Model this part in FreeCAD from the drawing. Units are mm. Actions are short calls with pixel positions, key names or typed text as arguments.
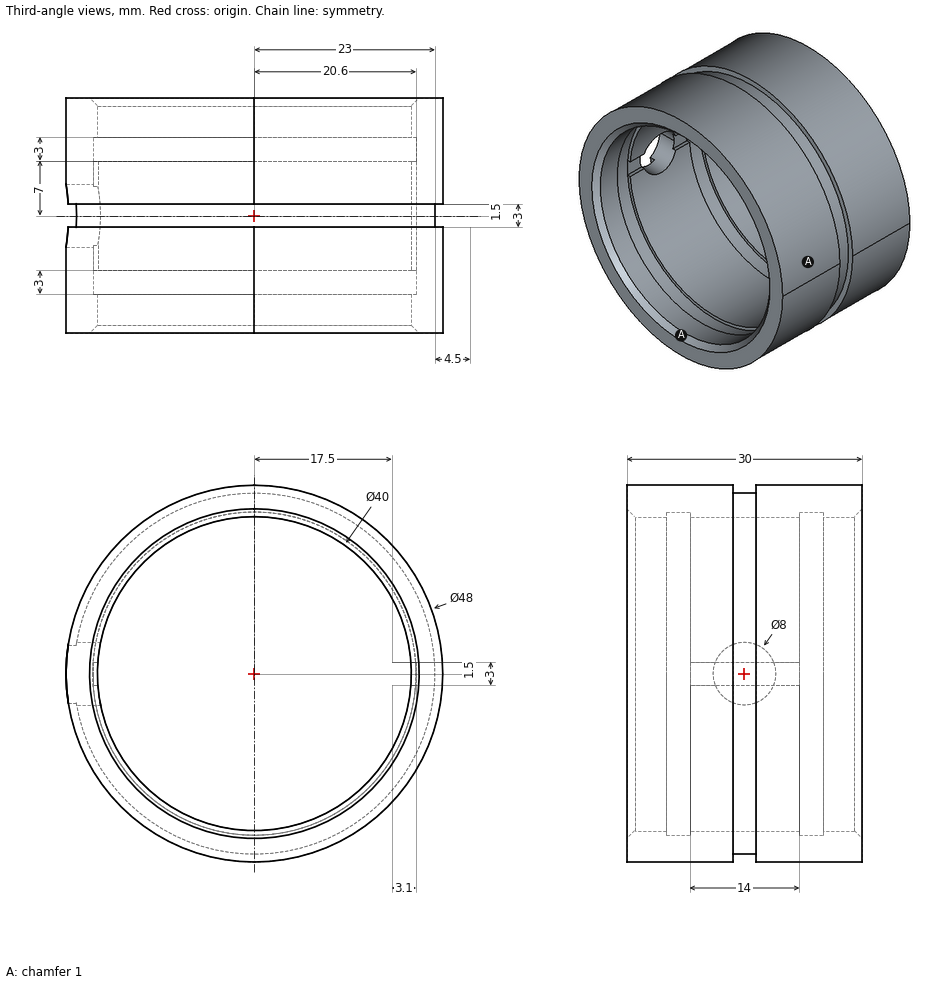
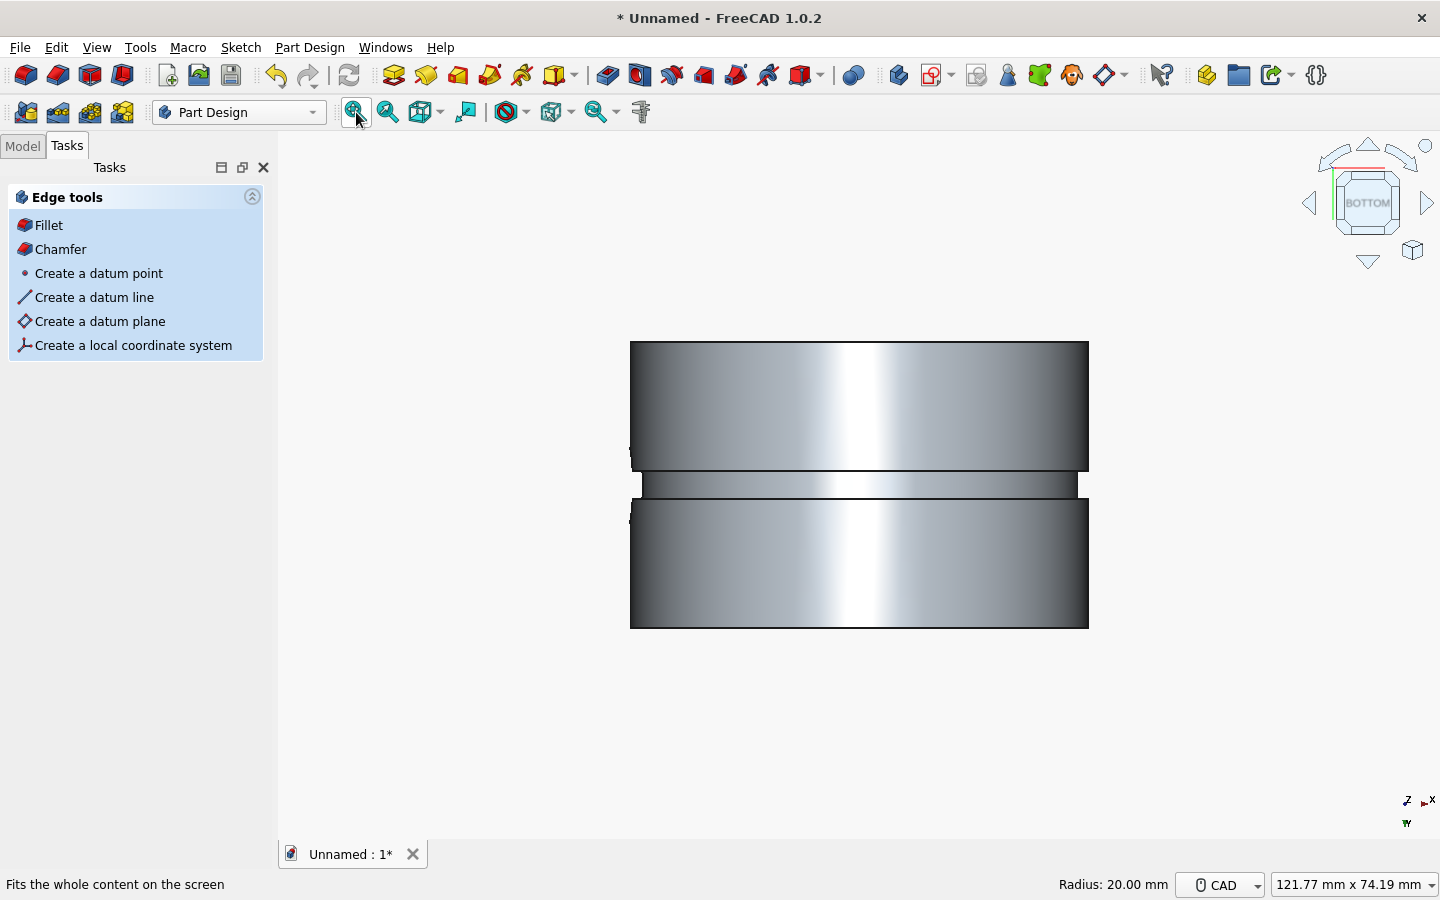
key(4)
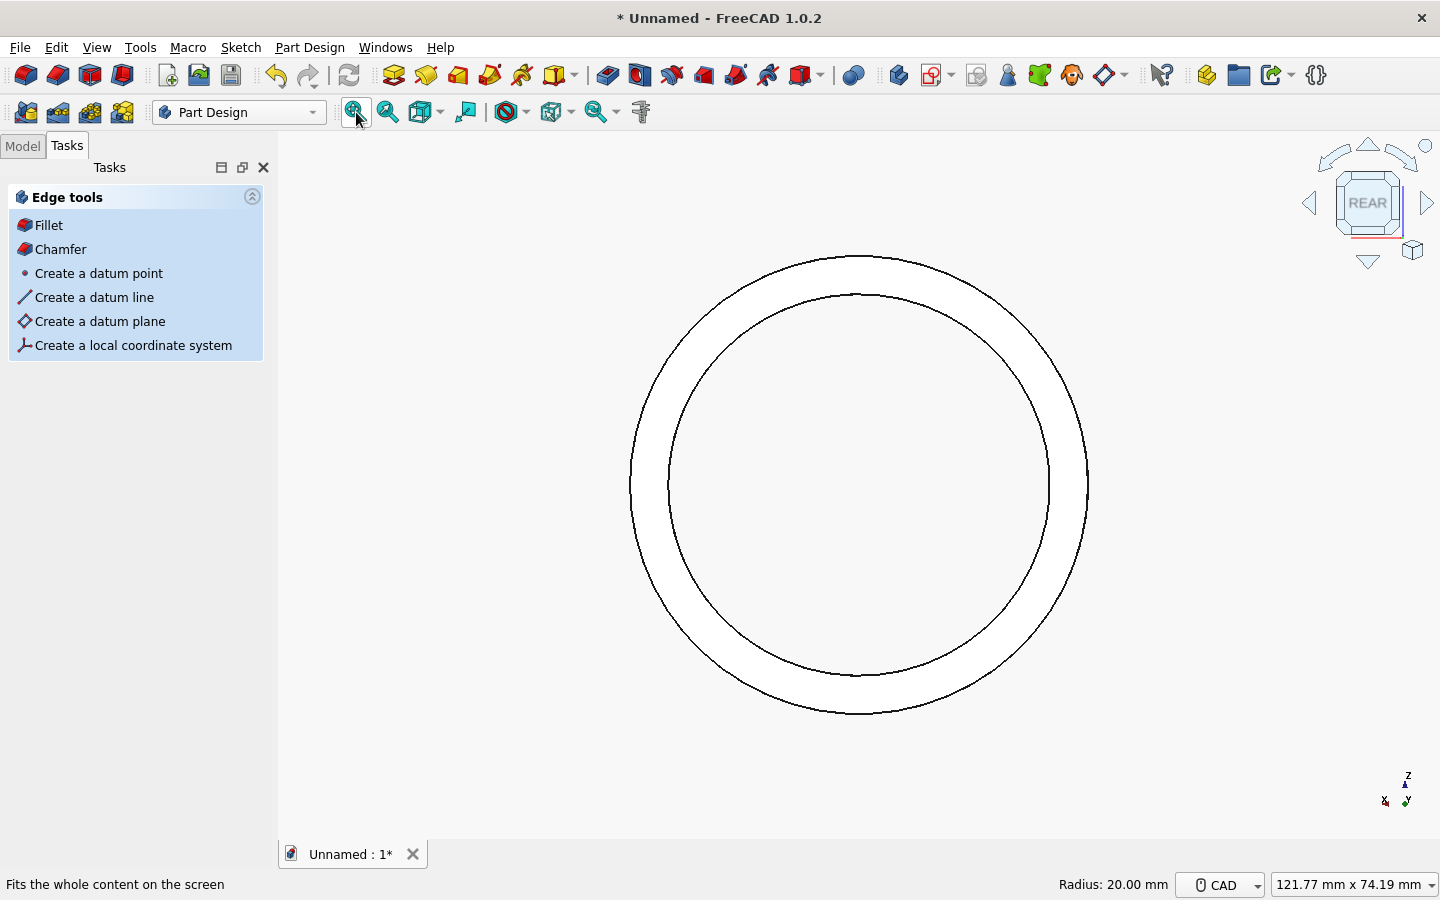
click(1050, 484, ctrl)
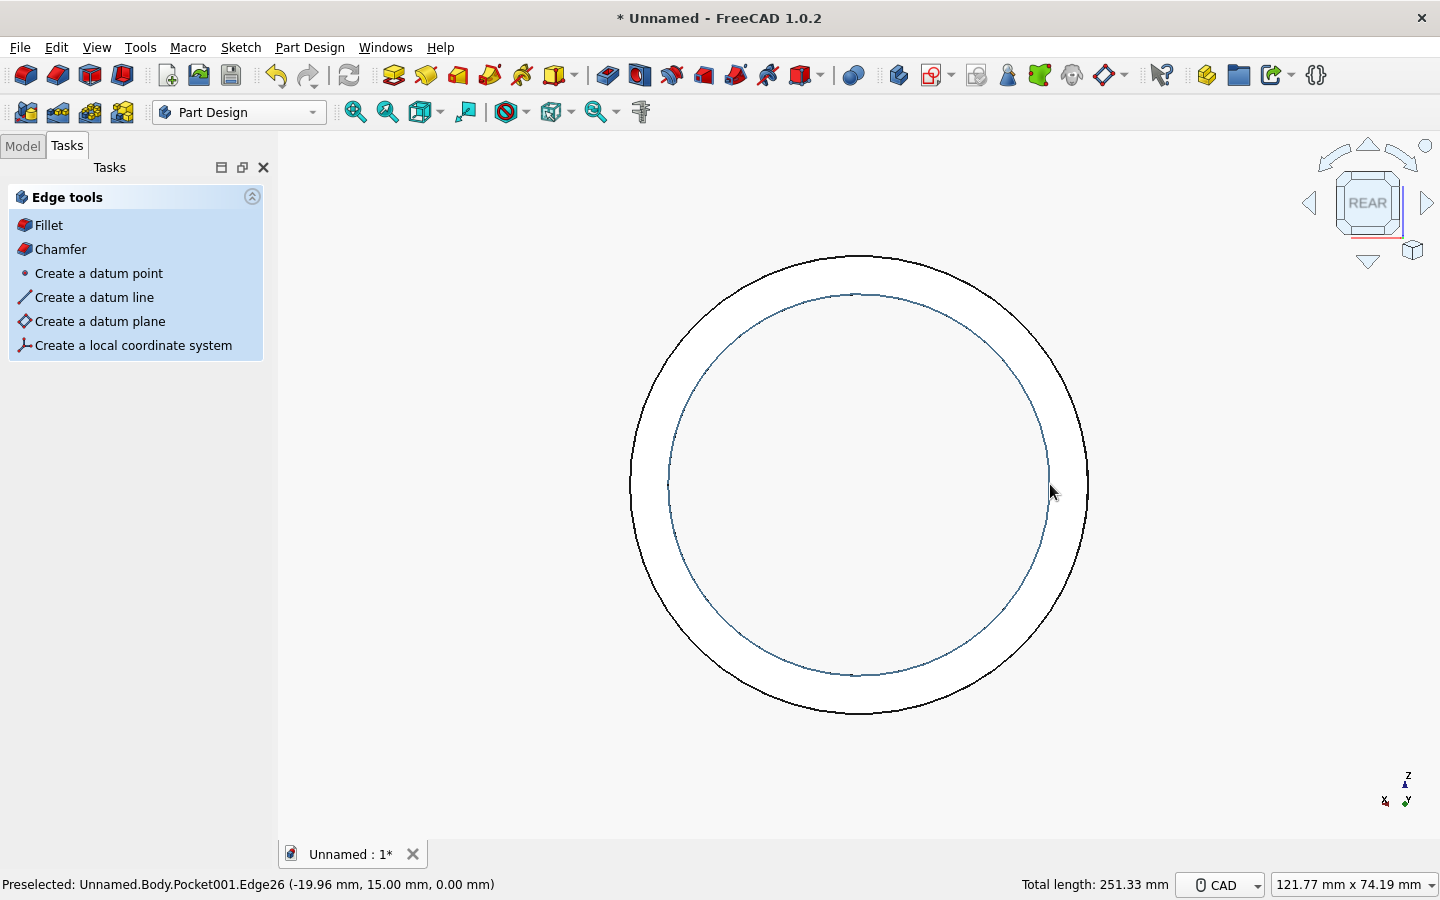
click(58, 76)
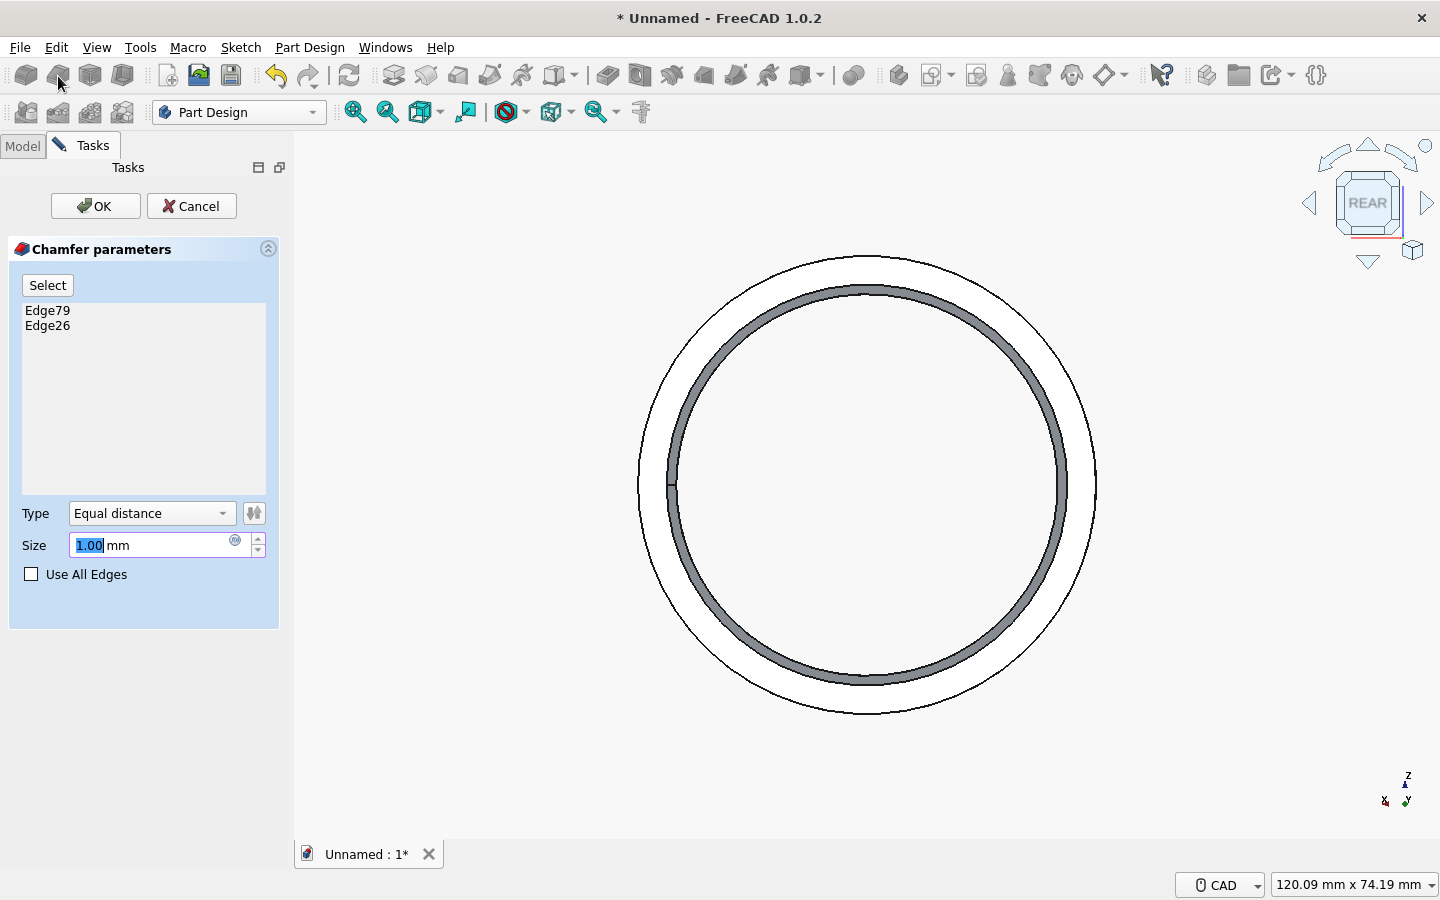
text(1)
key(Tab)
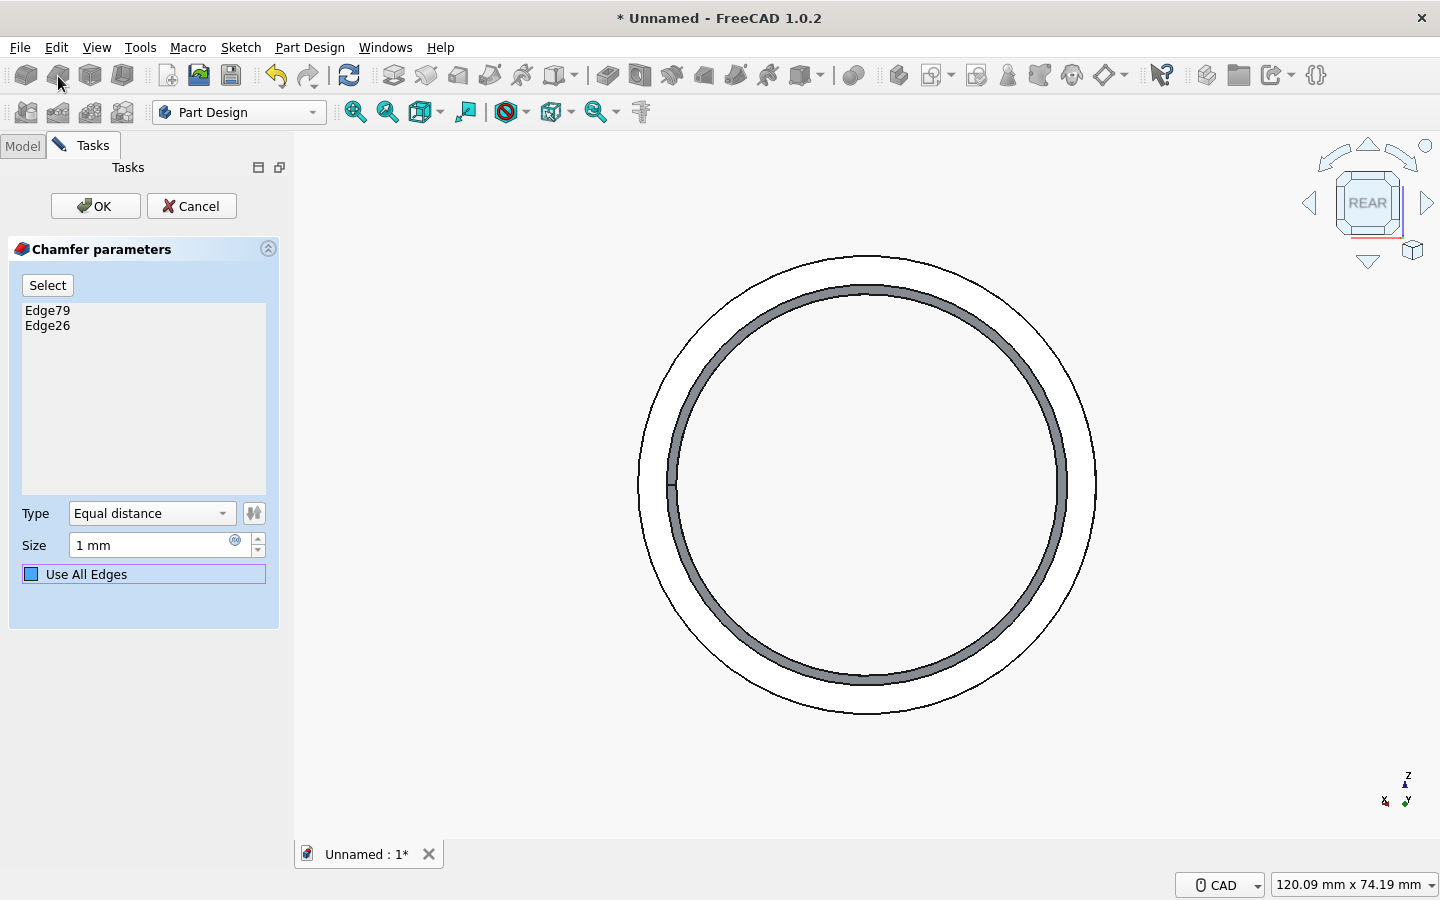
click(96, 206)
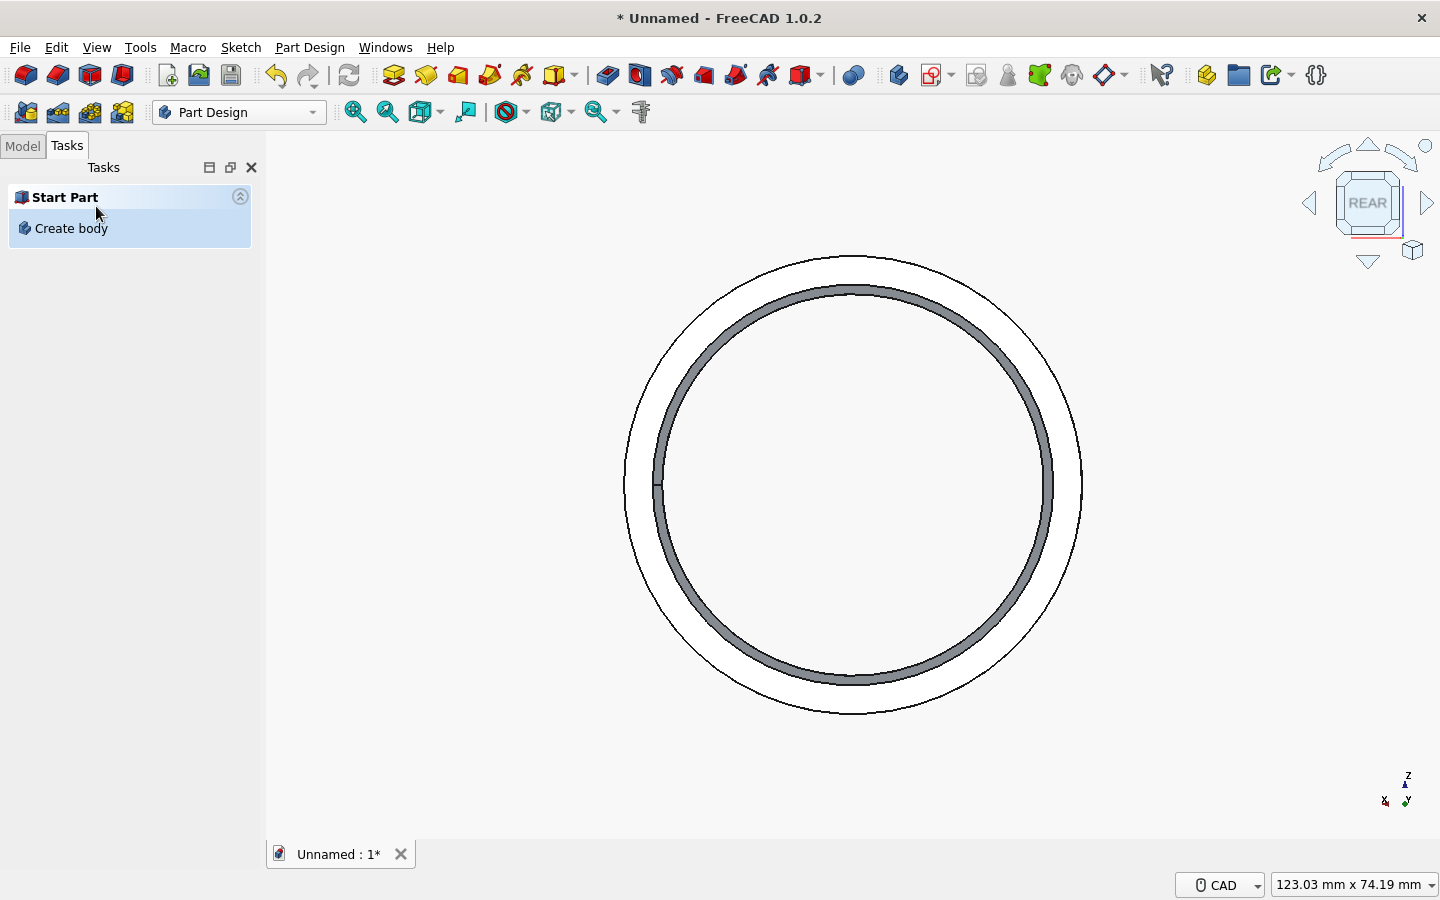
key(0)